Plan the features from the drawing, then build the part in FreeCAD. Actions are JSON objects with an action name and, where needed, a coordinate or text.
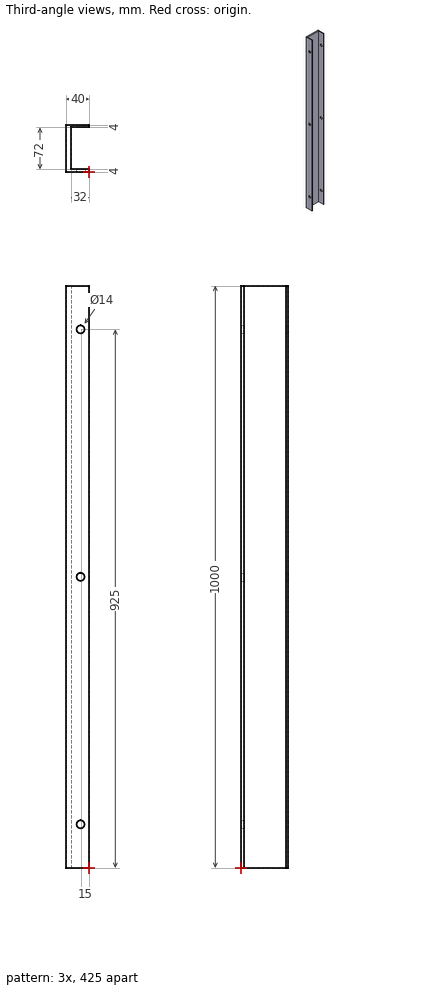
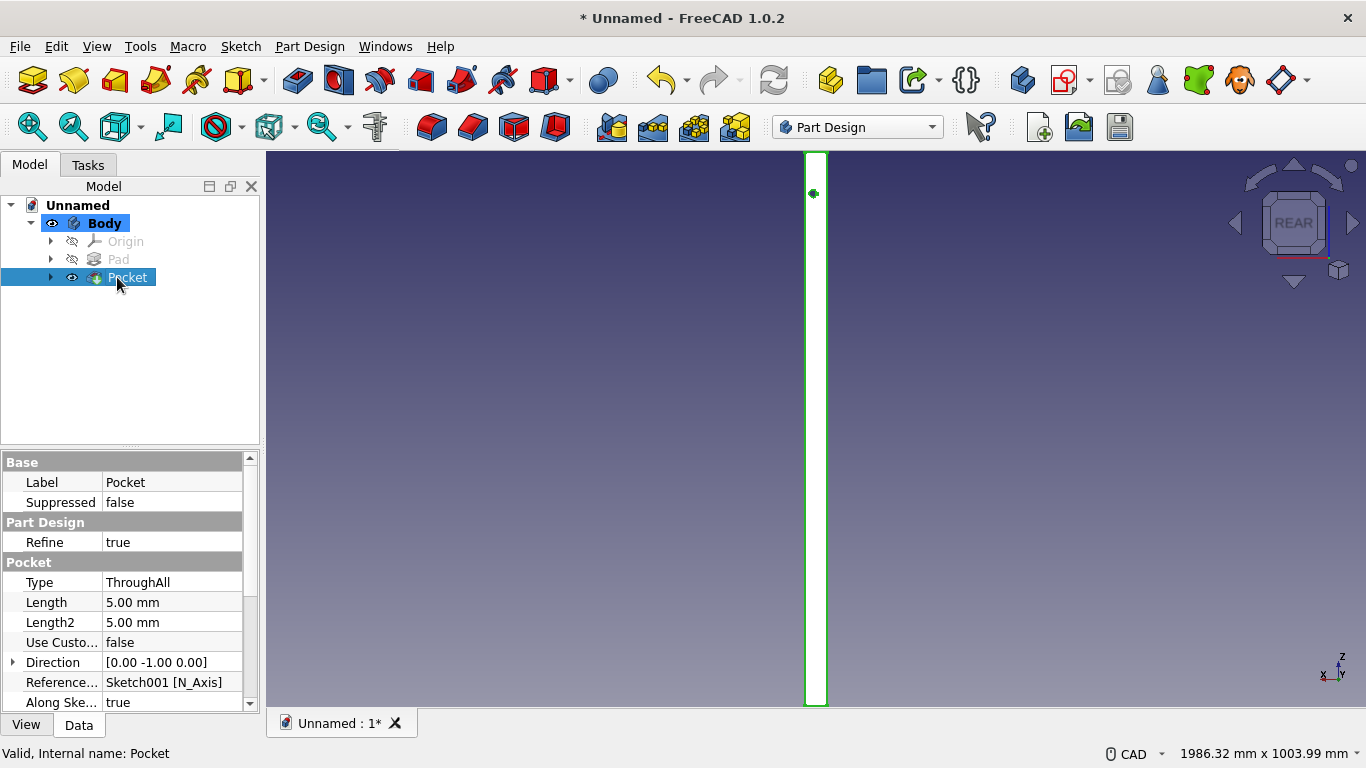
{"action": "left_click", "coordinate": [653, 128]}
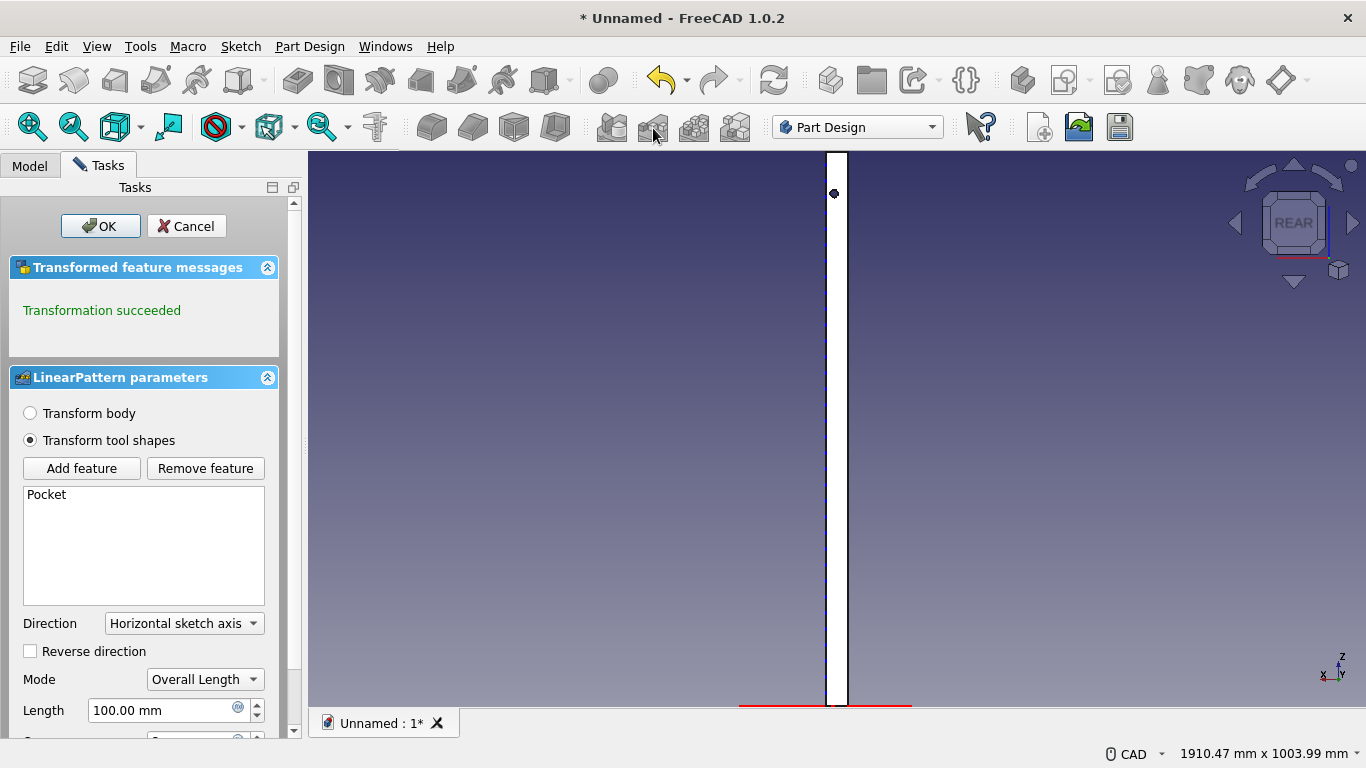
{"action": "left_click", "coordinate": [185, 624]}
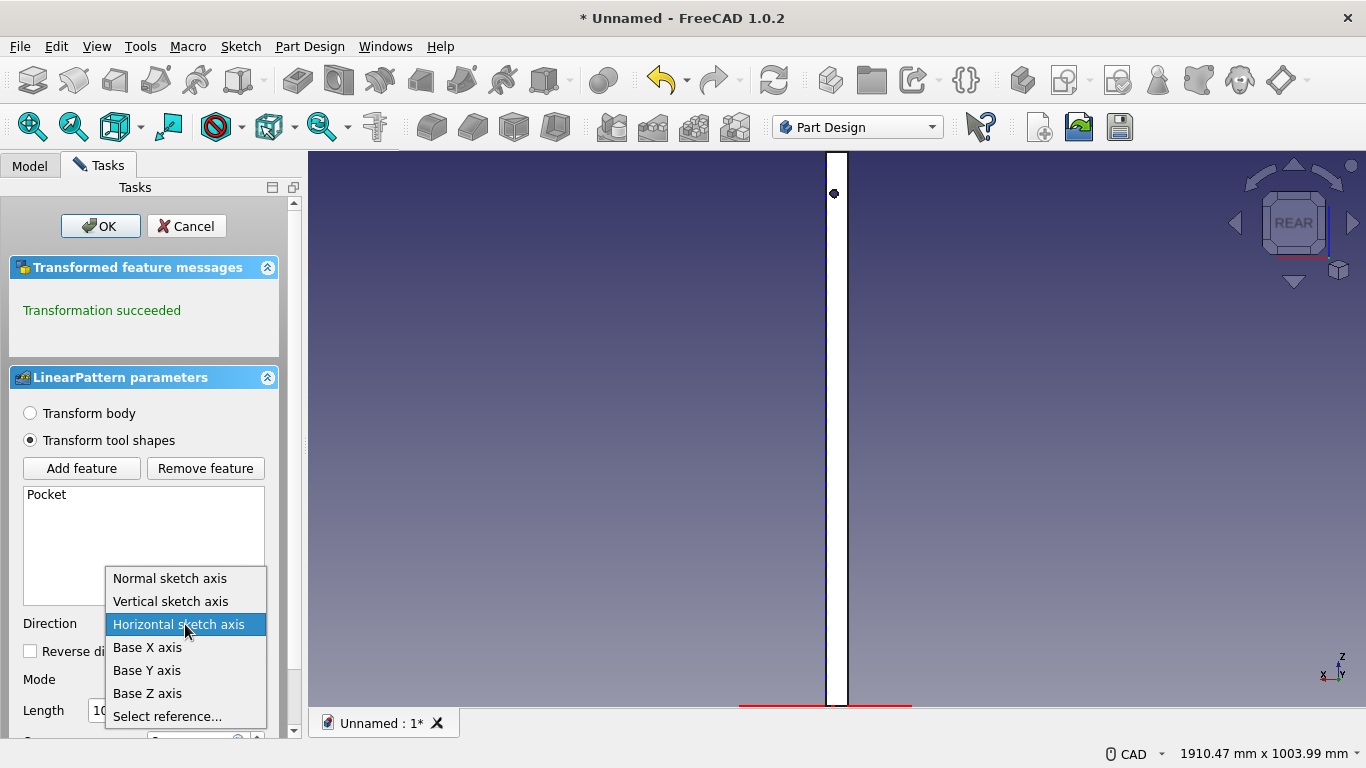
{"action": "left_click", "coordinate": [184, 694]}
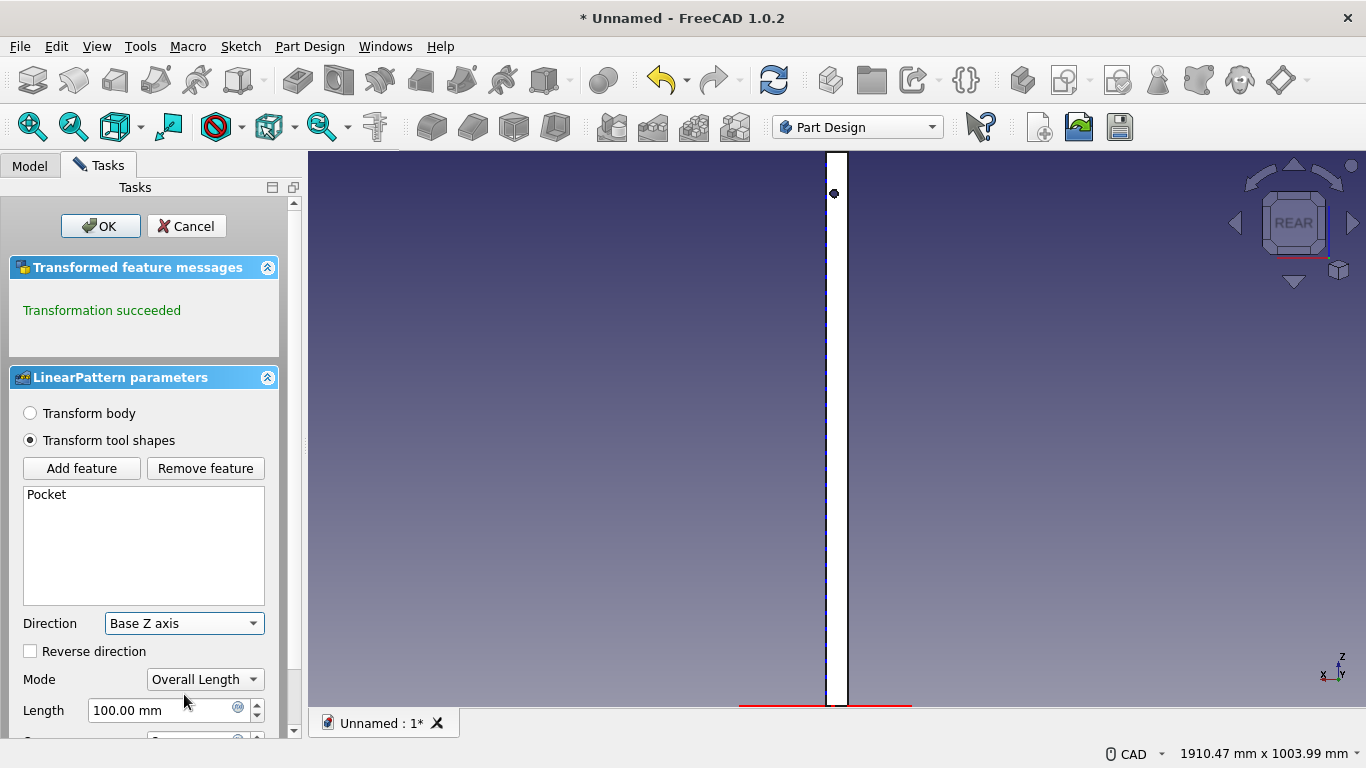
{"action": "left_click", "coordinate": [206, 680]}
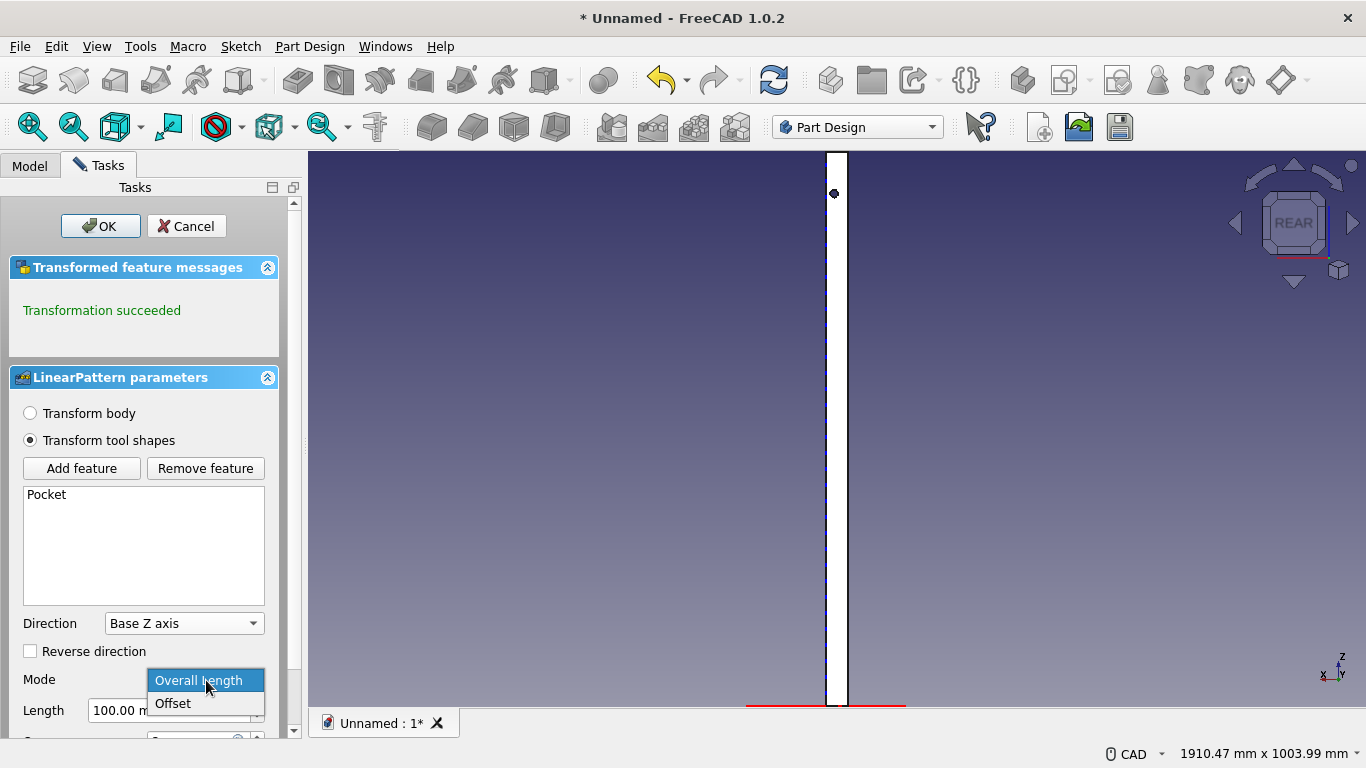
{"action": "left_click", "coordinate": [204, 704]}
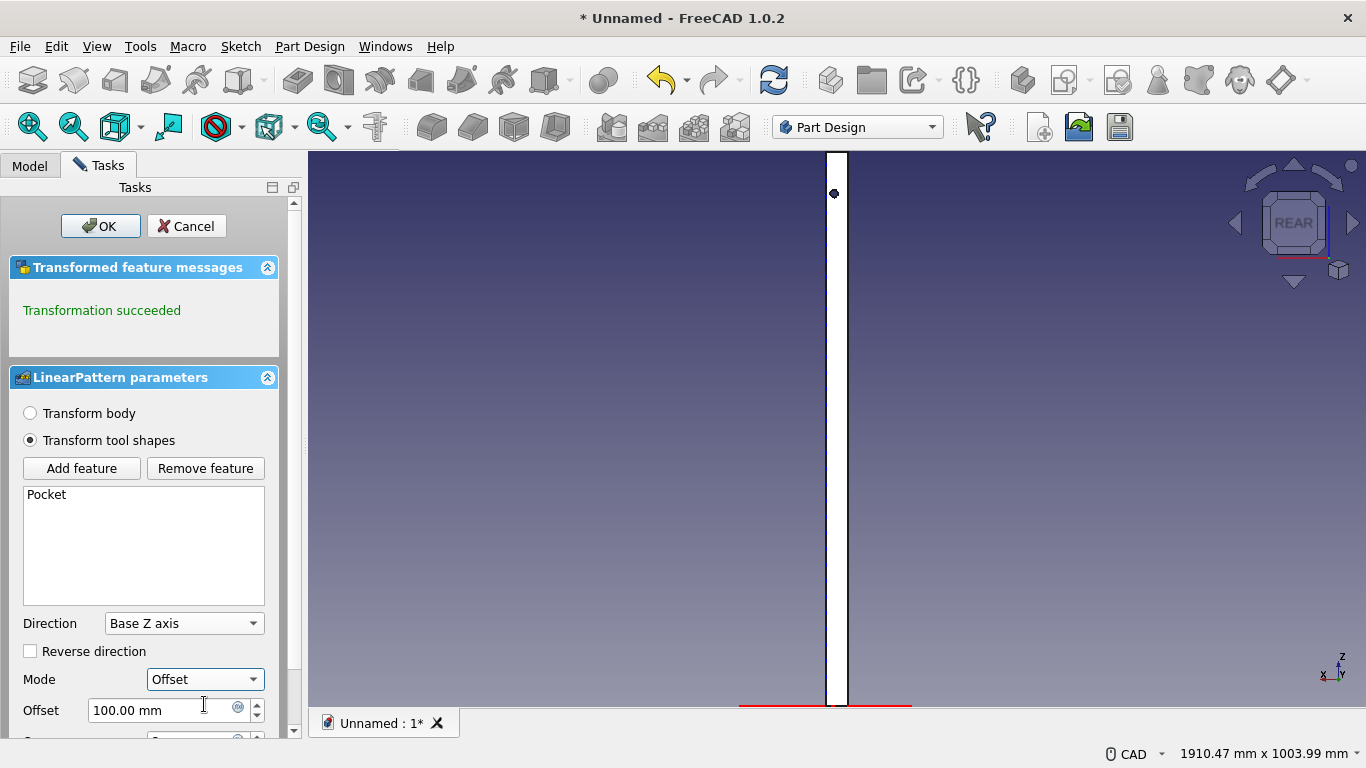
{"action": "triple_click", "coordinate": [170, 710]}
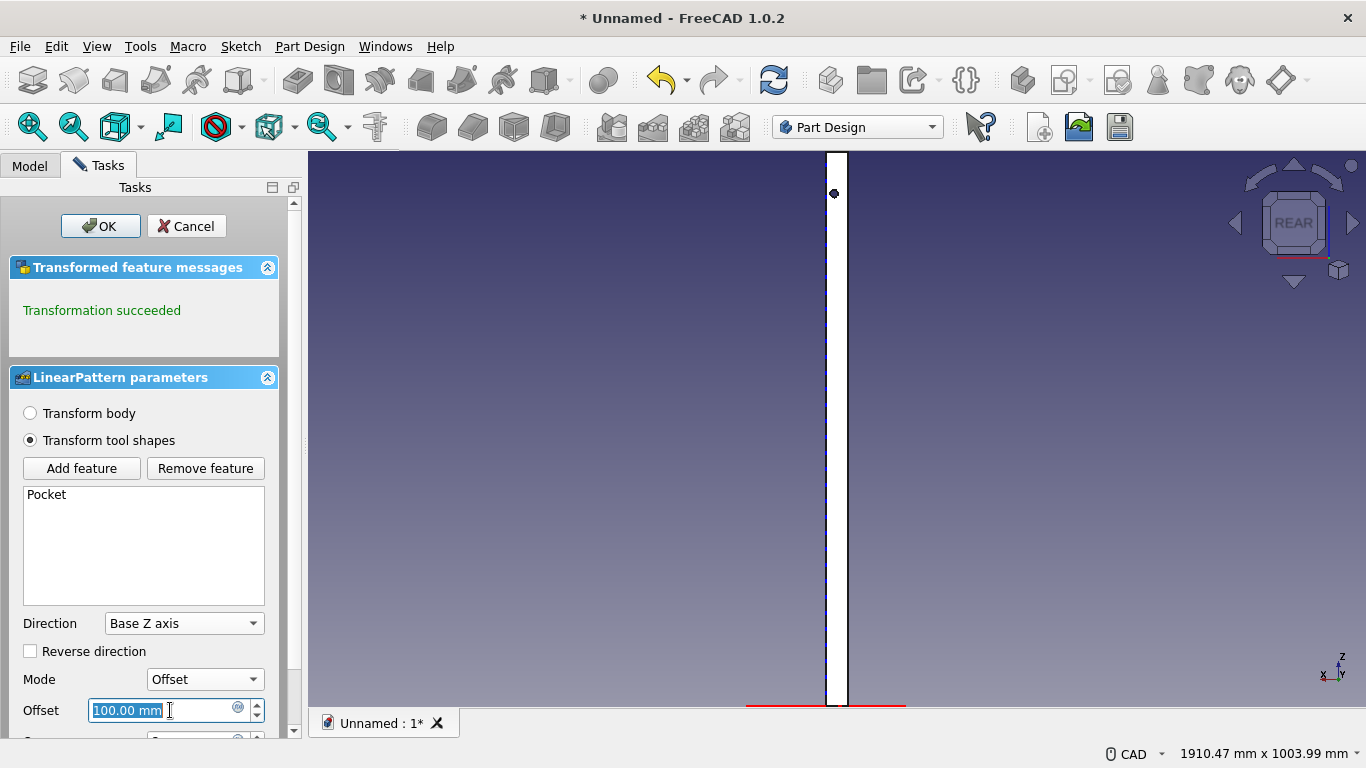
{"action": "type", "text": "425"}
{"action": "key", "text": "Tab"}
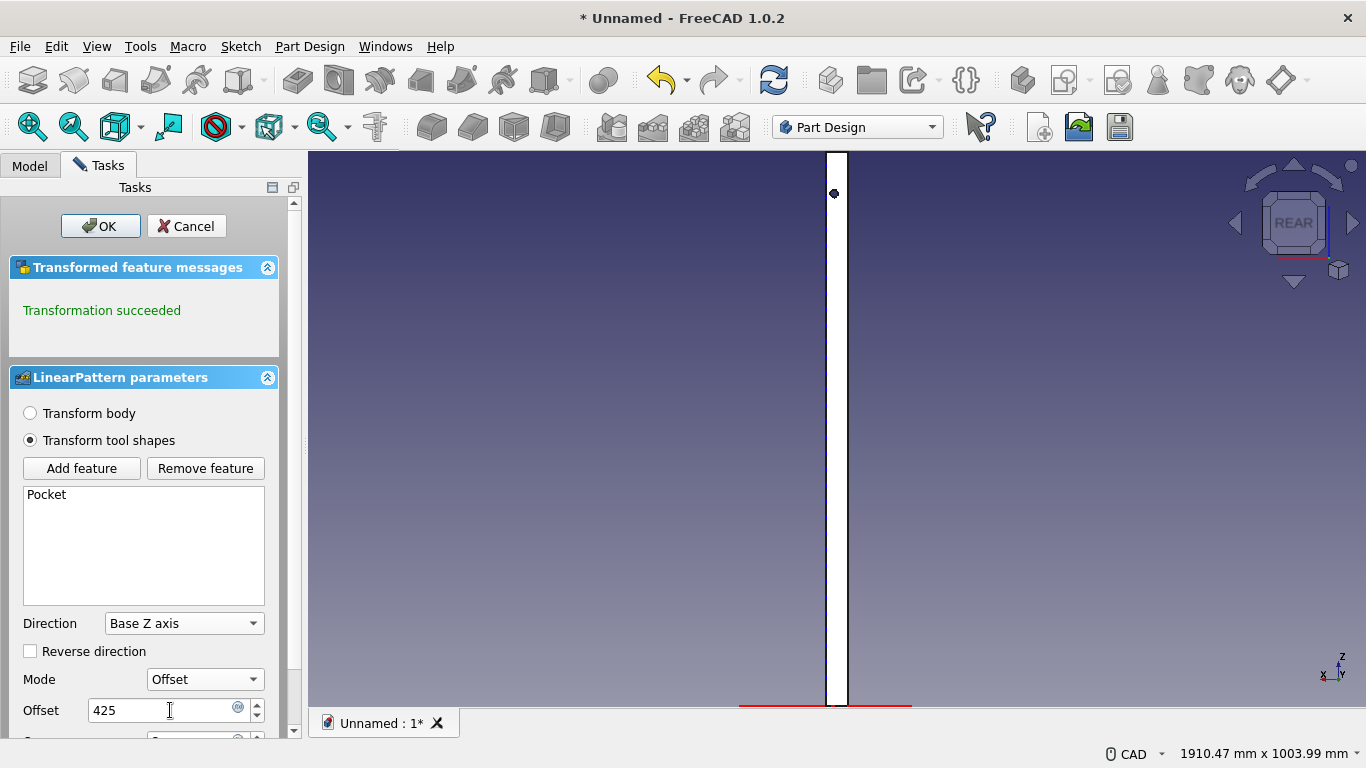
{"action": "scroll", "coordinate": [294, 468], "scroll_direction": "down", "scroll_amount": 2}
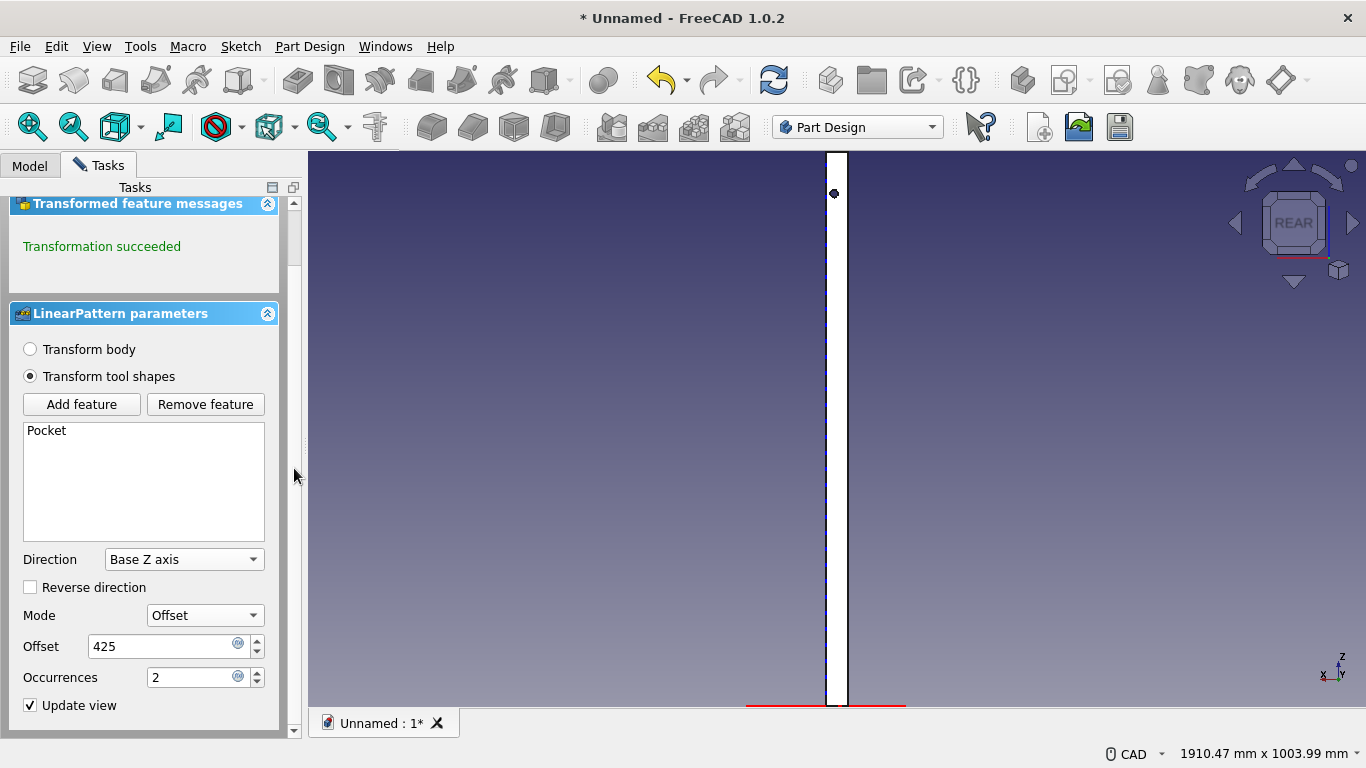
{"action": "triple_click", "coordinate": [199, 678]}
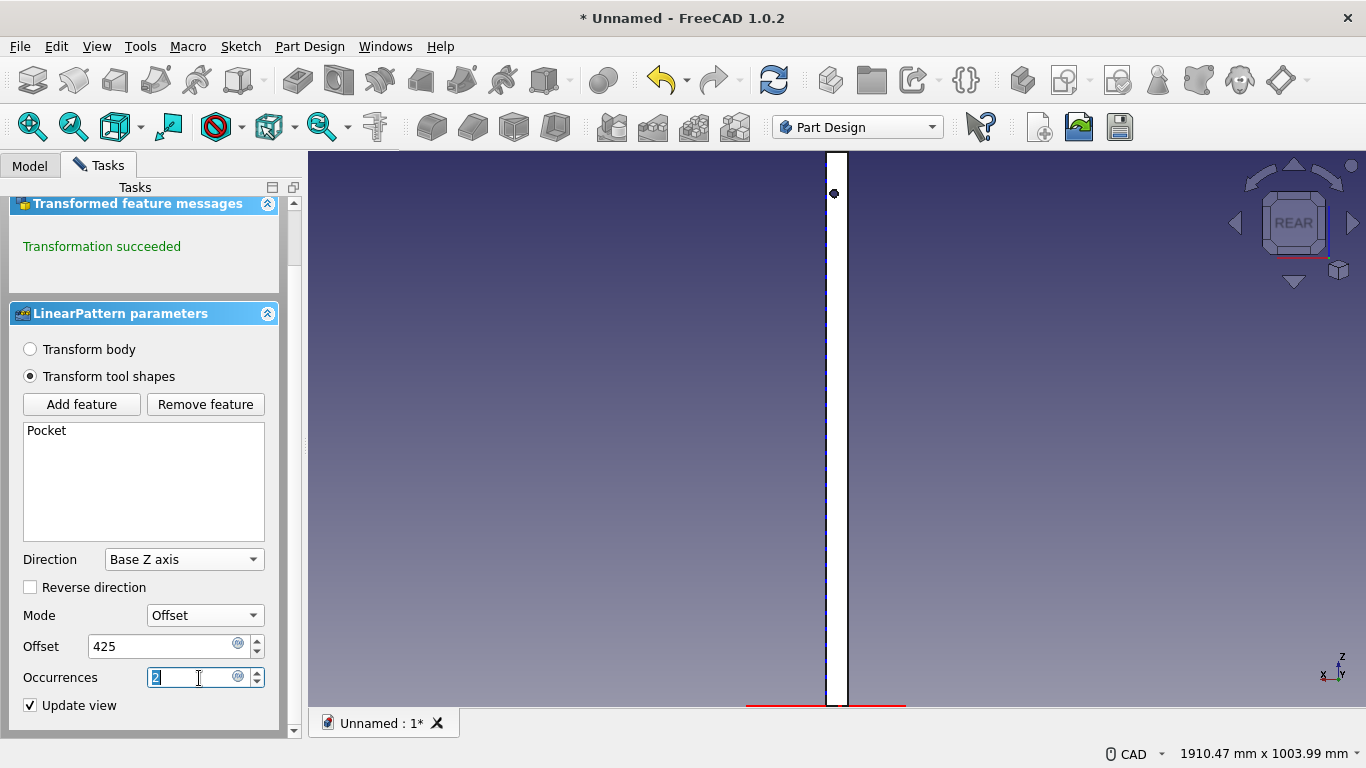
{"action": "type", "text": "3"}
{"action": "key", "text": "Tab"}